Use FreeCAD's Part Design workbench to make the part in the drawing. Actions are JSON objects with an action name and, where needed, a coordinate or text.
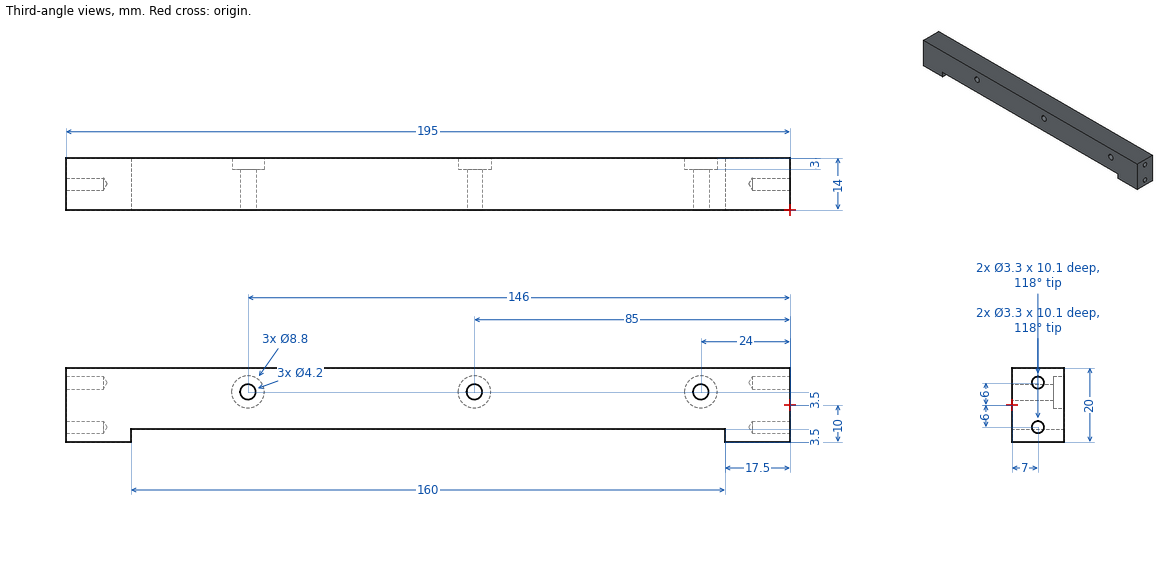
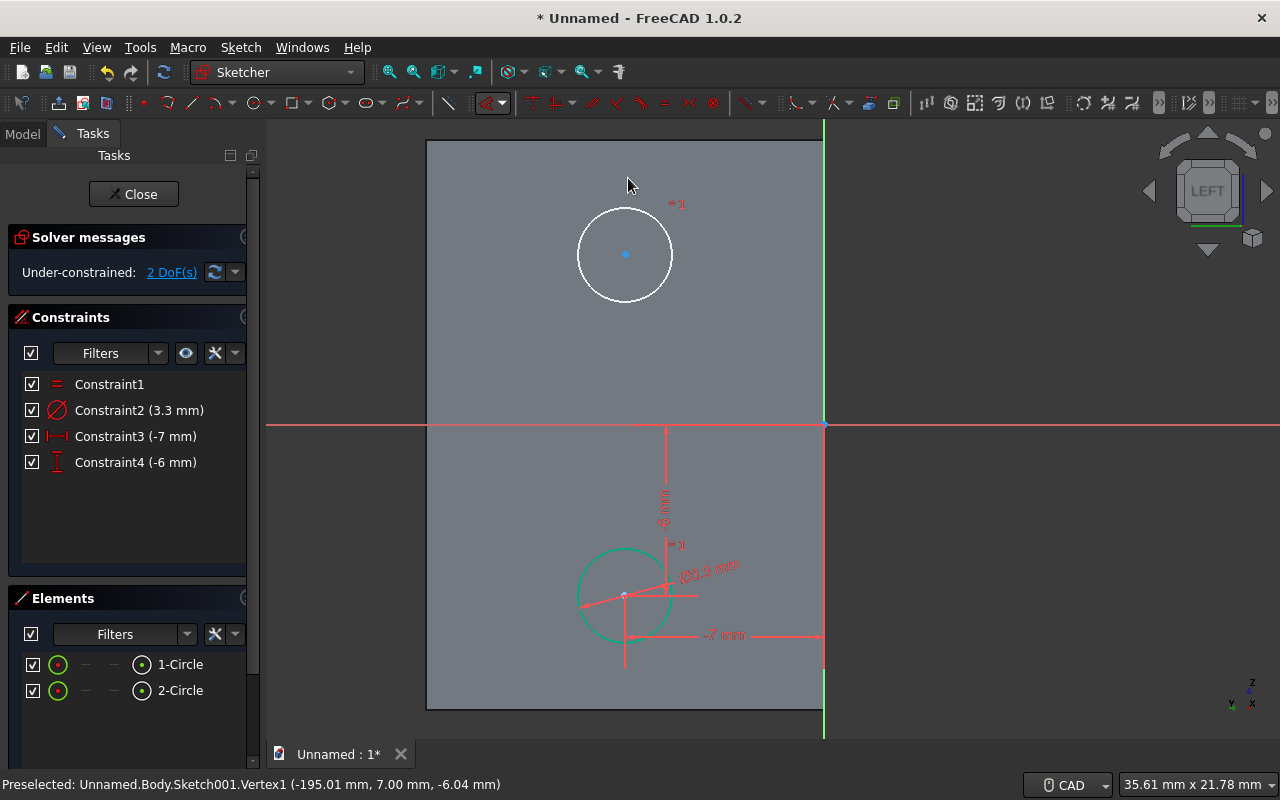
{"action": "left_click", "coordinate": [625, 255]}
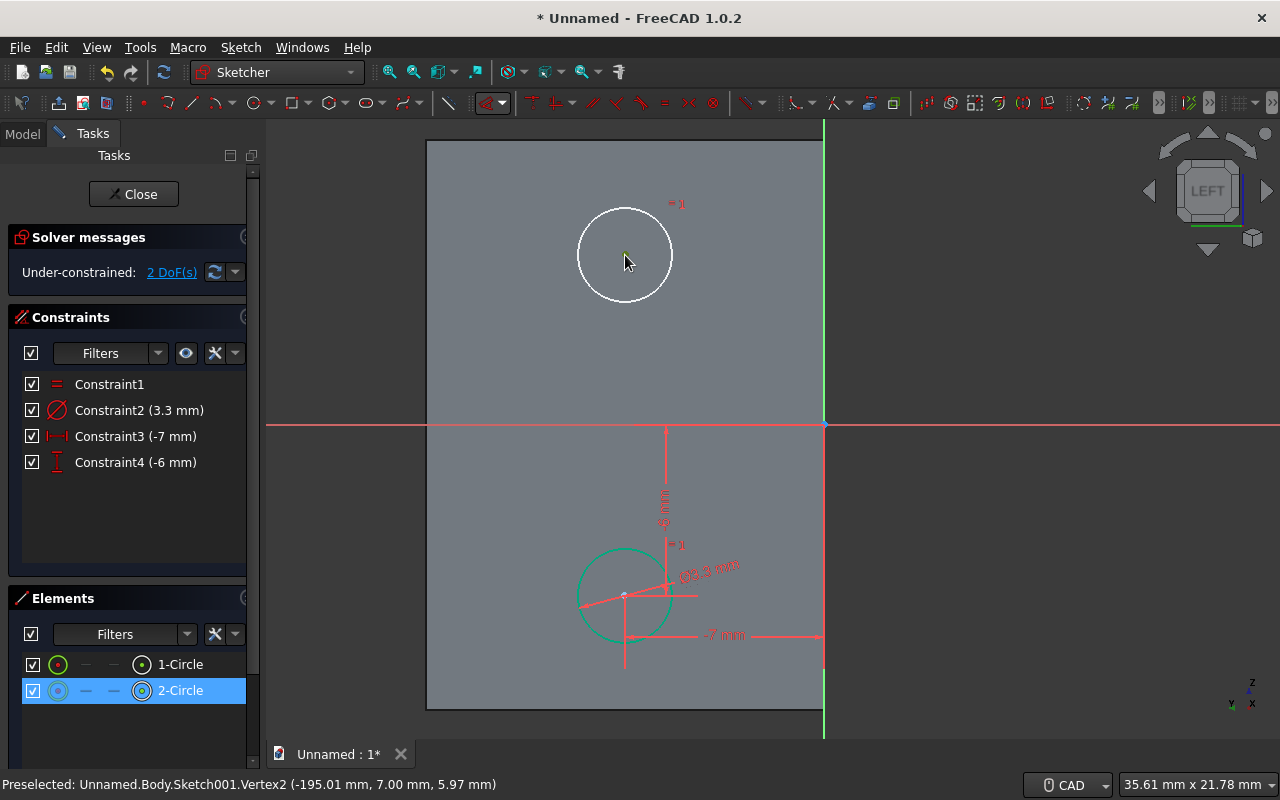
{"action": "key", "text": "l"}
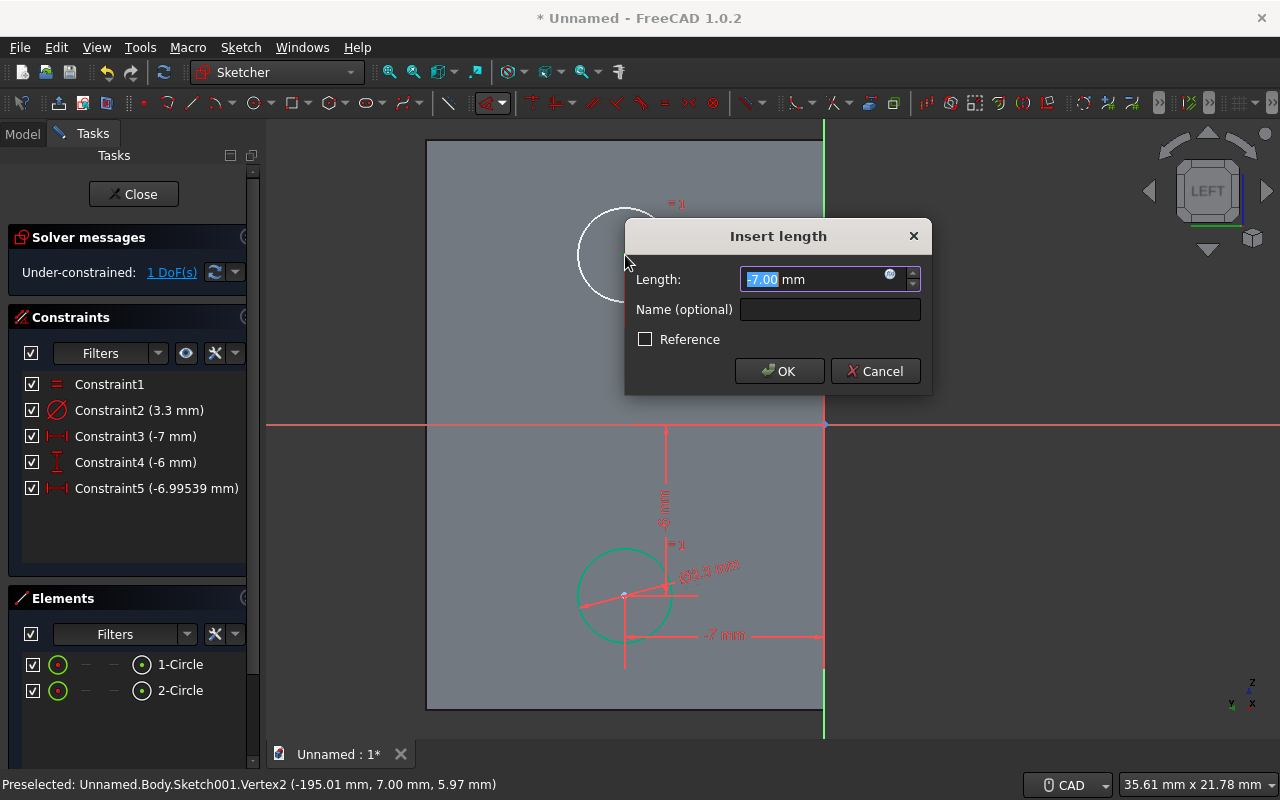
{"action": "type", "text": "-7"}
{"action": "key", "text": "Return"}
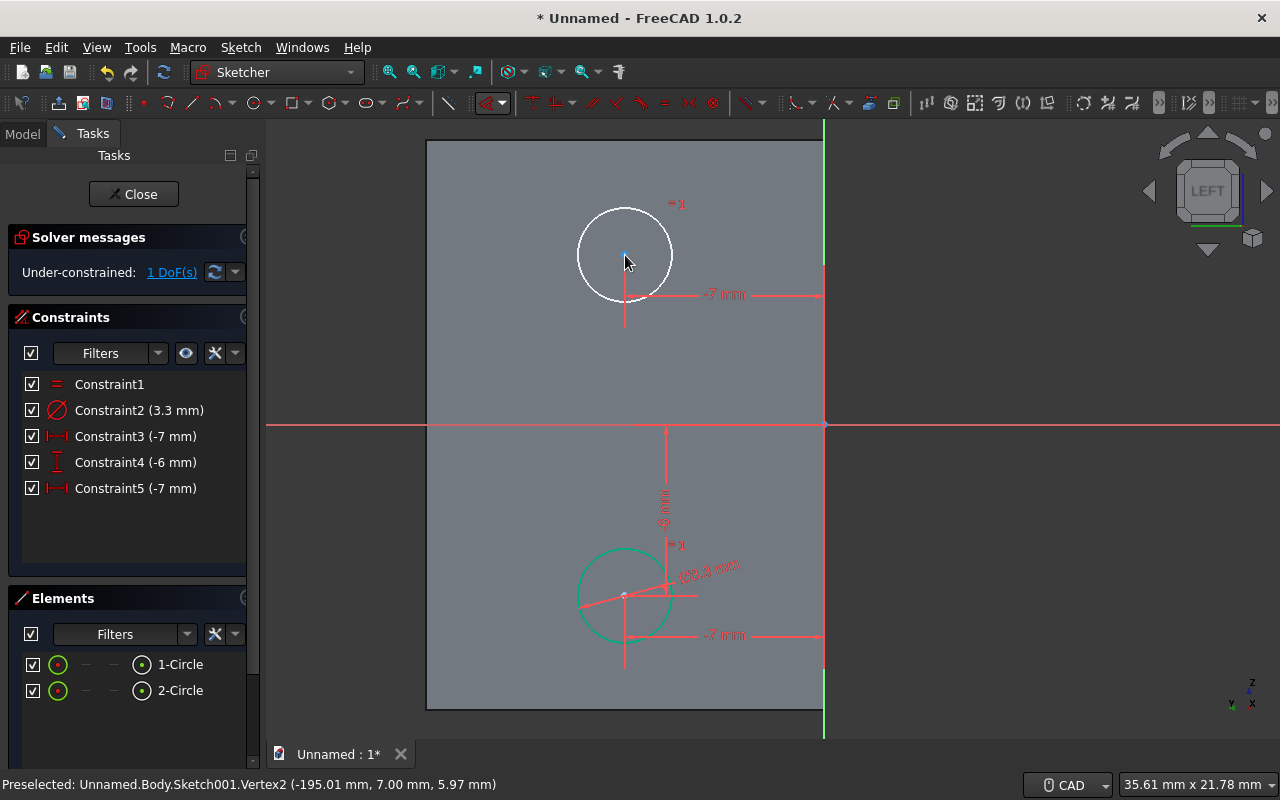
{"action": "left_click", "coordinate": [625, 255]}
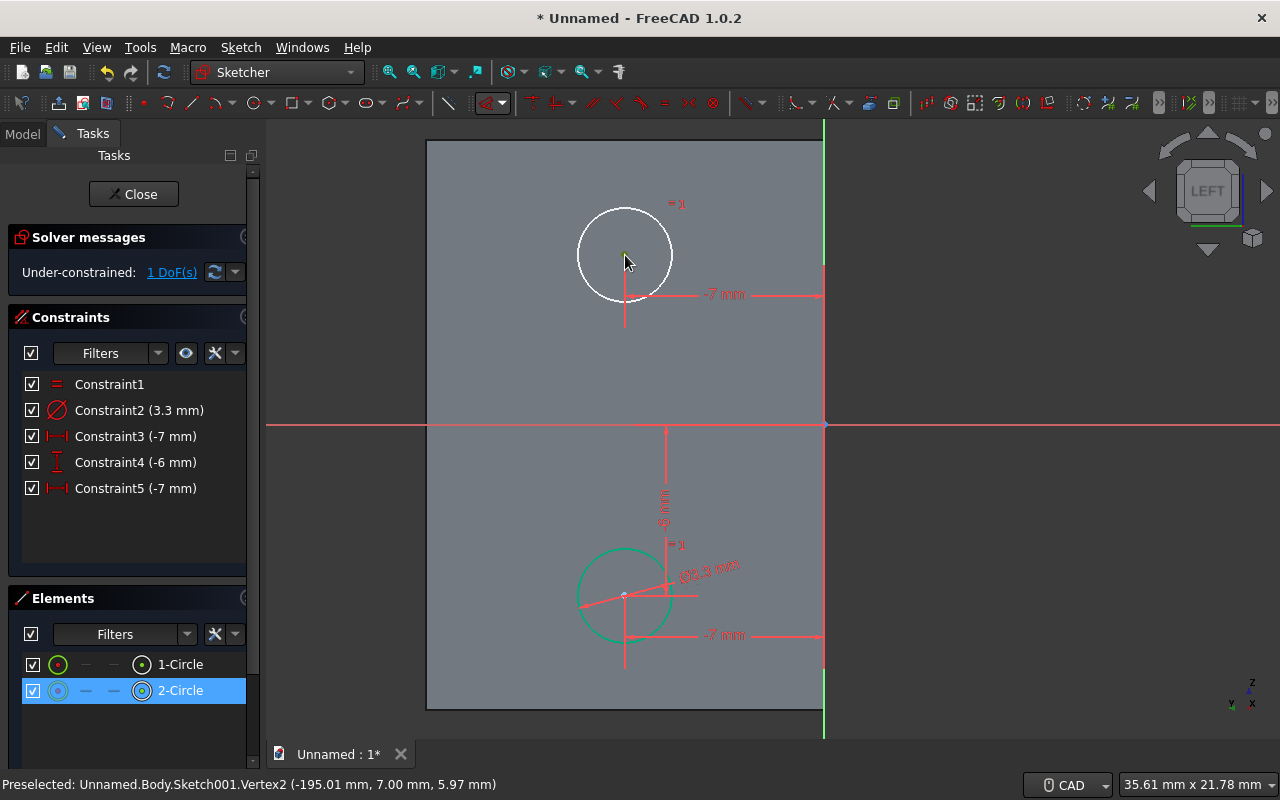
{"action": "left_click", "coordinate": [504, 104]}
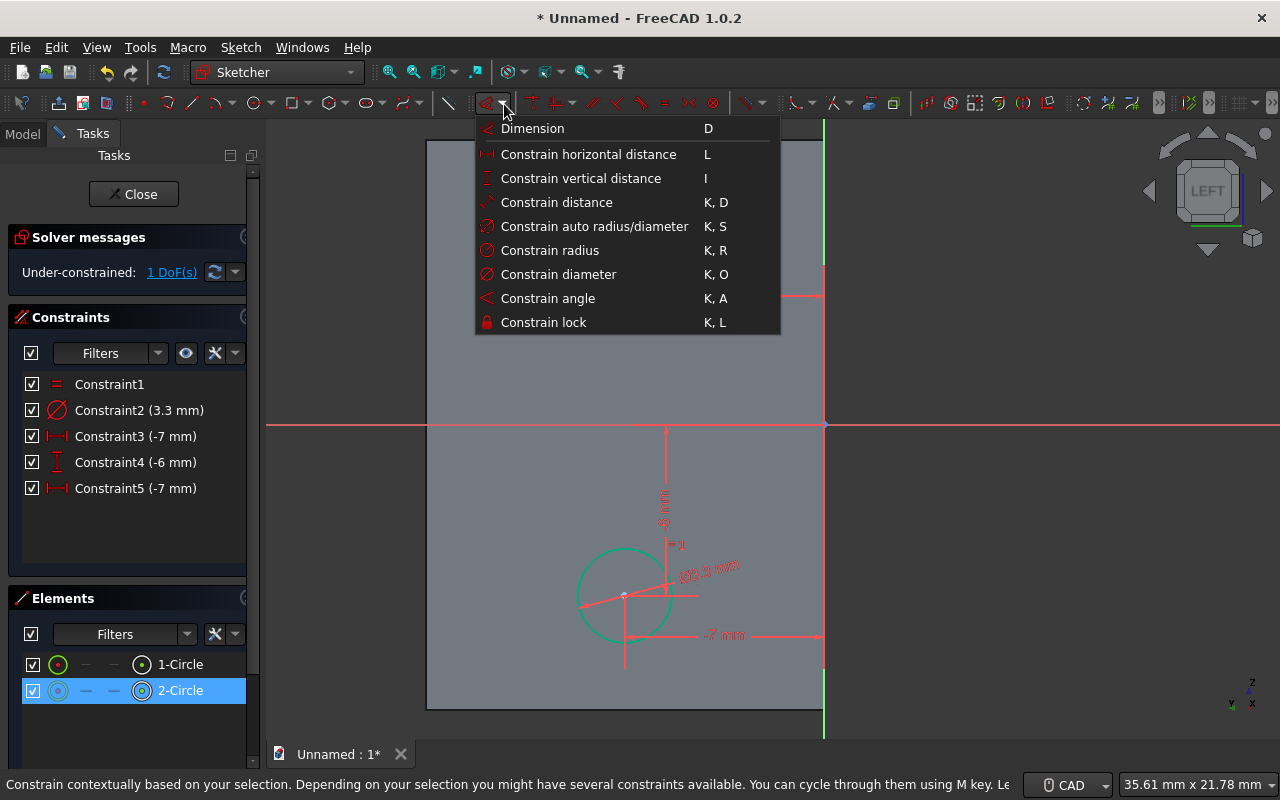
{"action": "left_click", "coordinate": [628, 178]}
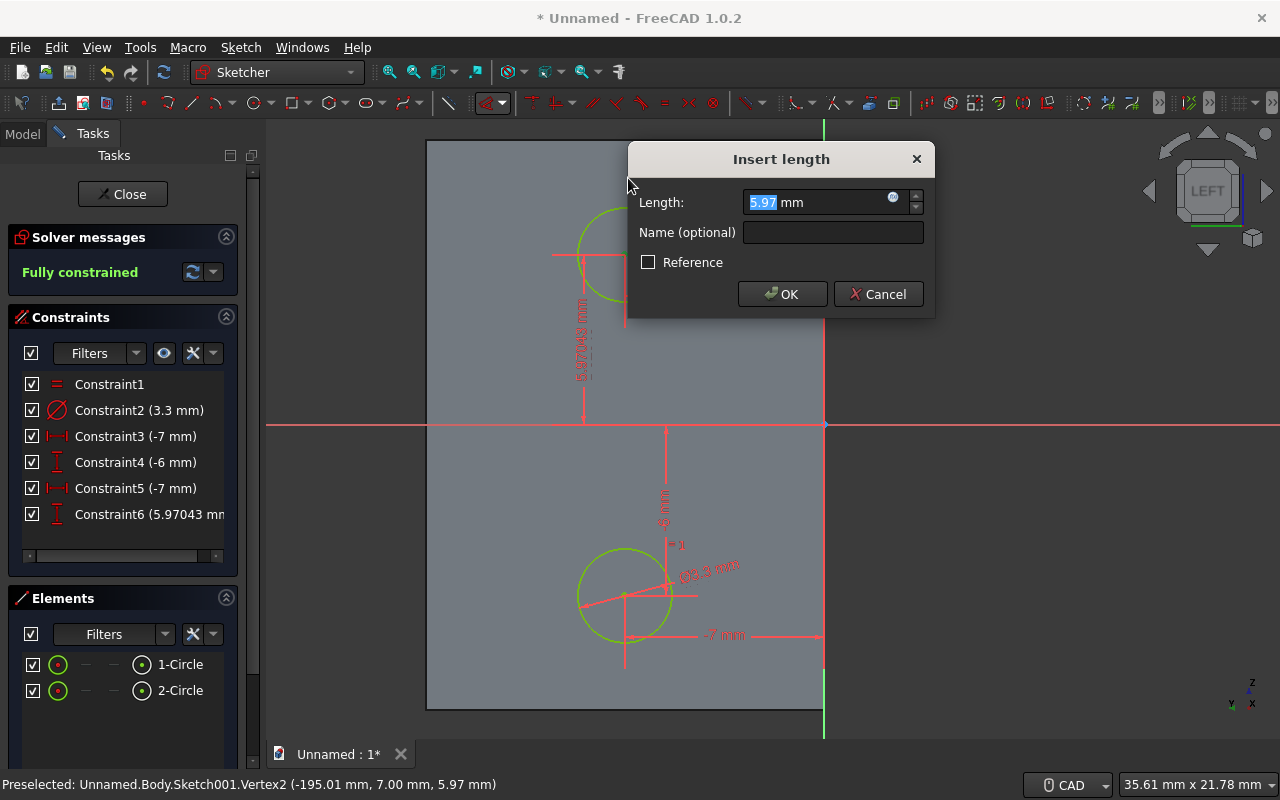
{"action": "type", "text": "6"}
{"action": "key", "text": "Return"}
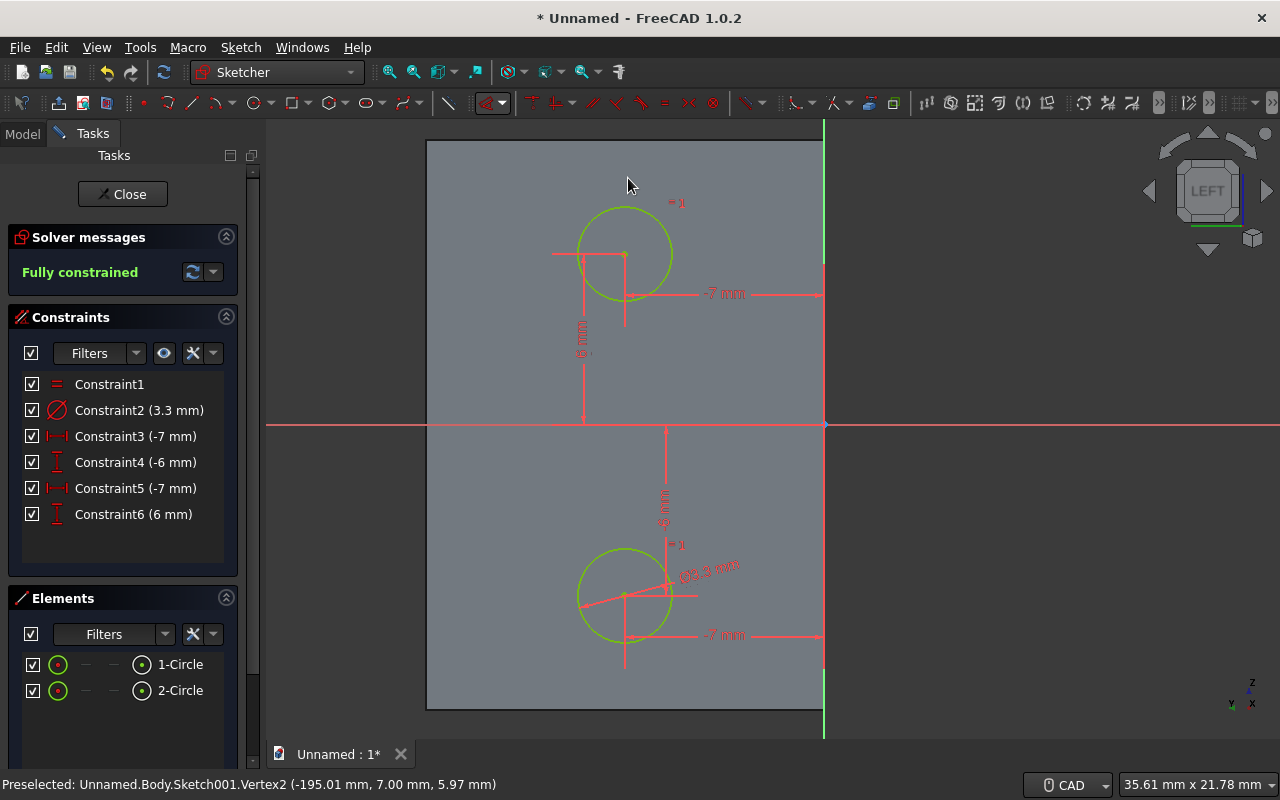
{"action": "left_click", "coordinate": [123, 194]}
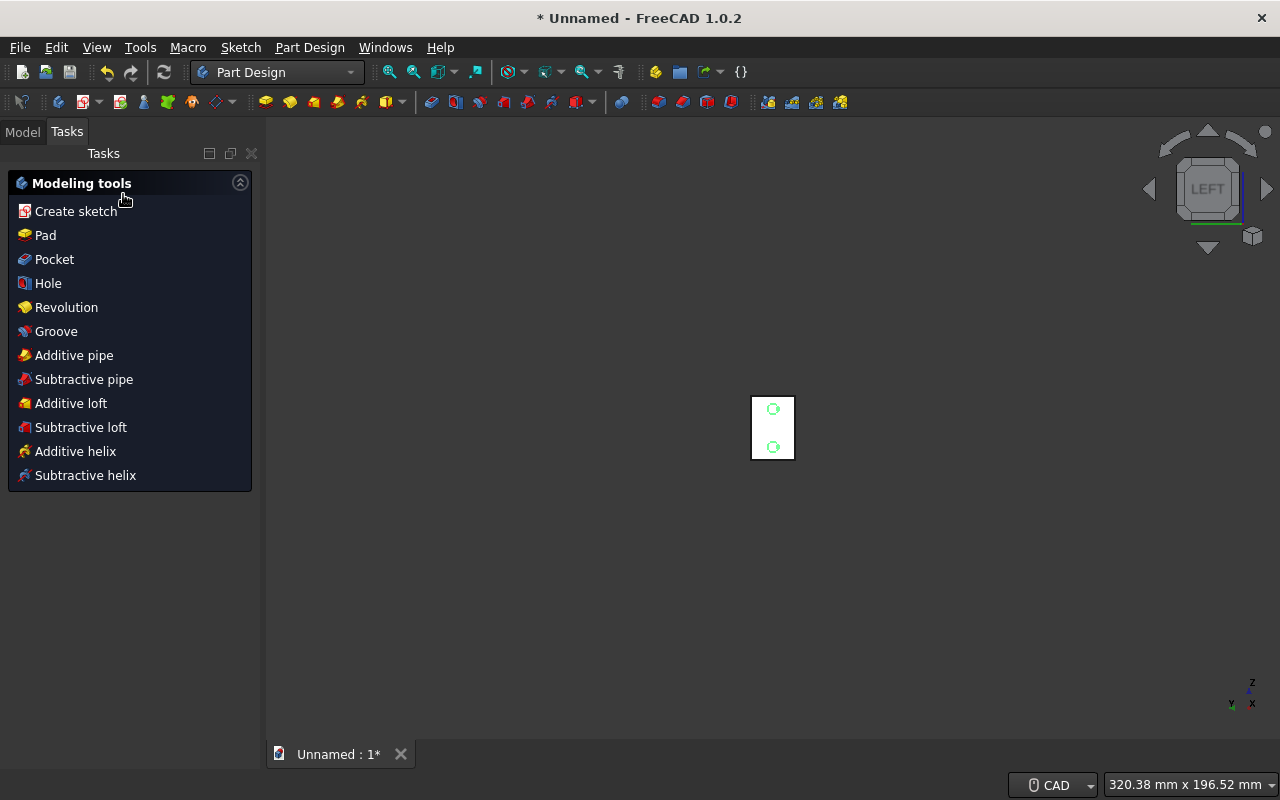
{"action": "left_click", "coordinate": [456, 102]}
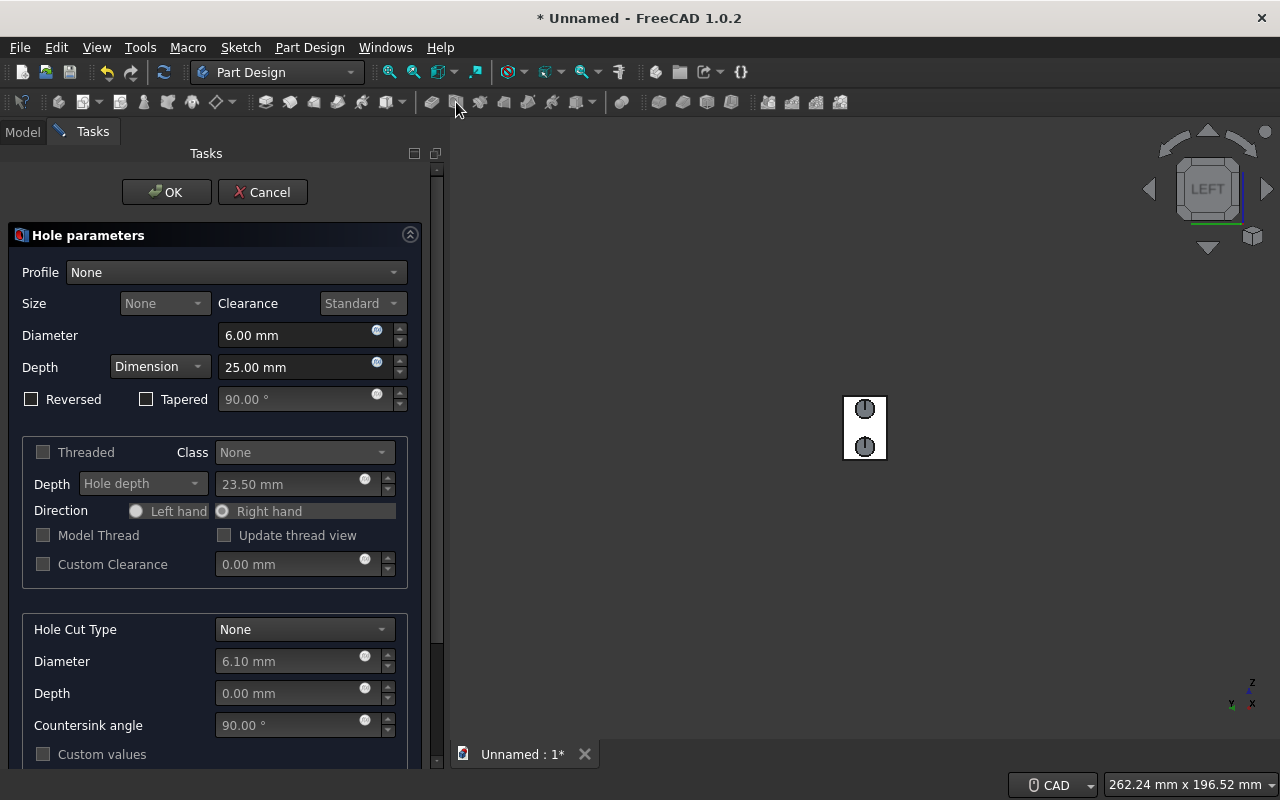
{"action": "triple_click", "coordinate": [305, 335]}